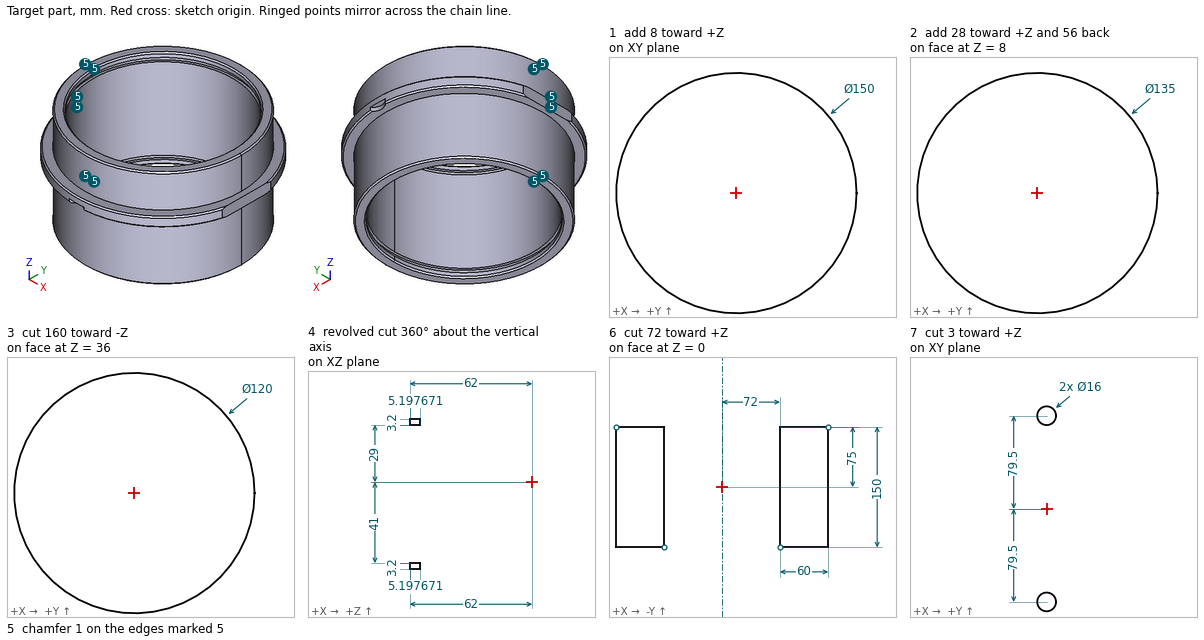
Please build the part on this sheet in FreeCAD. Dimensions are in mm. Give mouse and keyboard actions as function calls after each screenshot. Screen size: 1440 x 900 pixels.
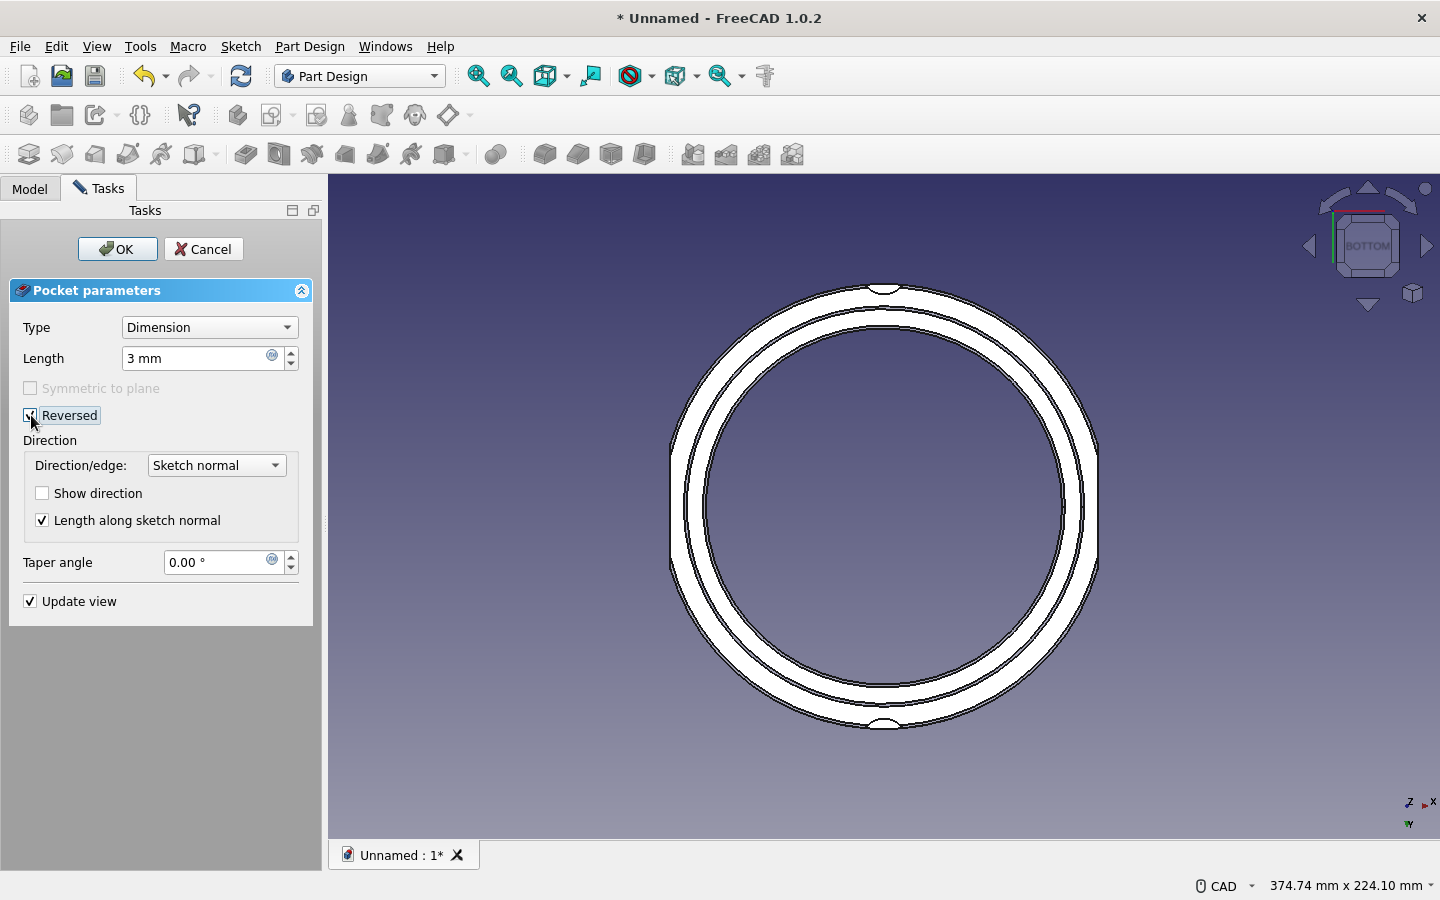
click(118, 249)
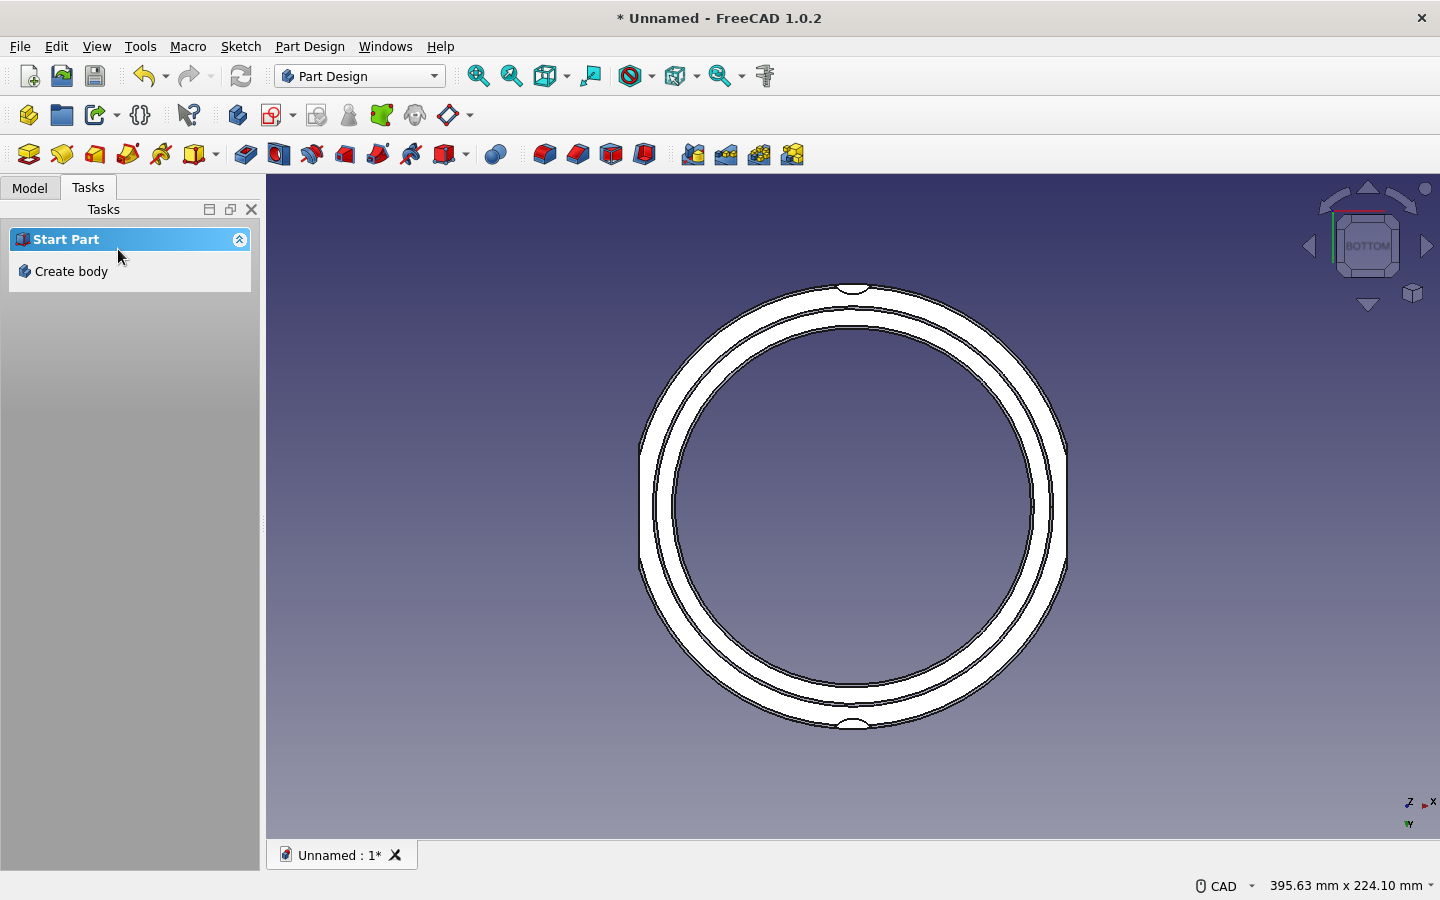
key(0)